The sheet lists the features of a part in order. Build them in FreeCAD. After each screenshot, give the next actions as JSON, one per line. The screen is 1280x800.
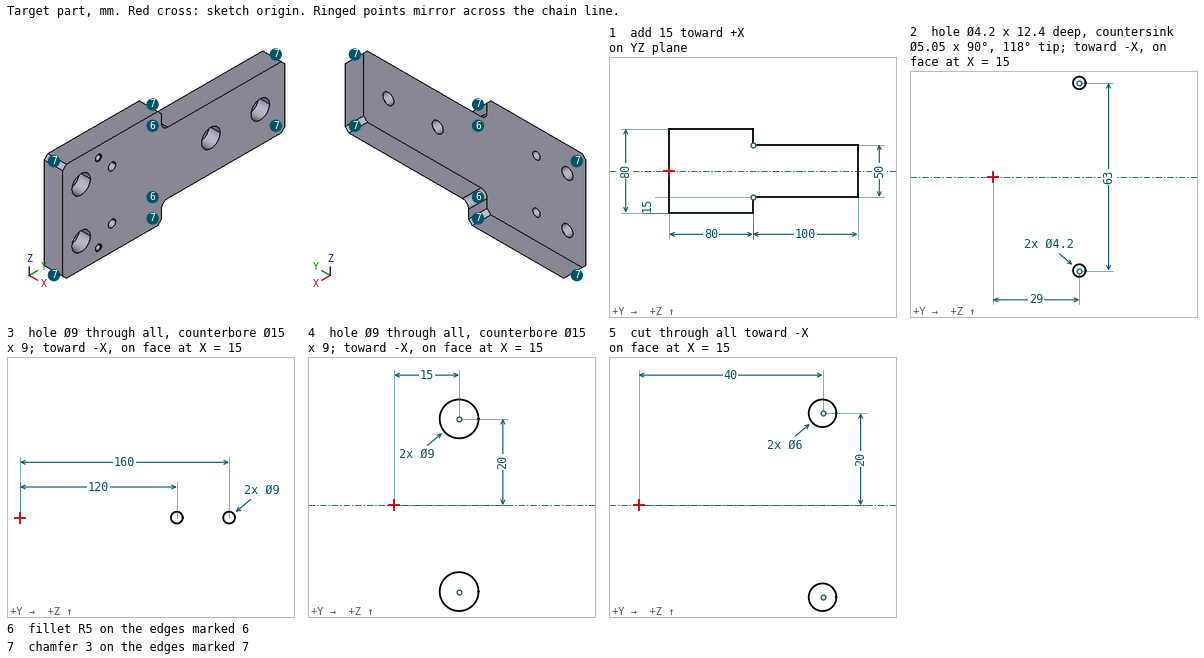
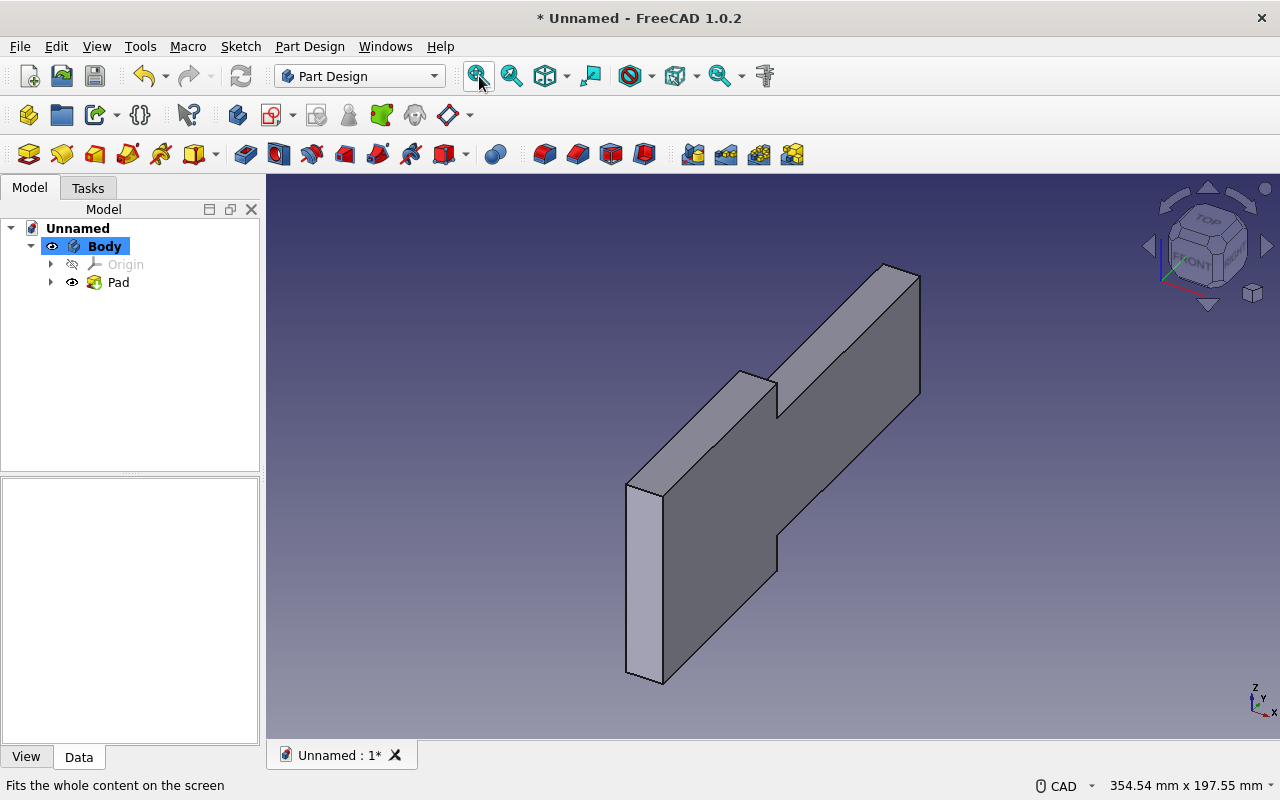
{"action": "left_click", "coordinate": [718, 535]}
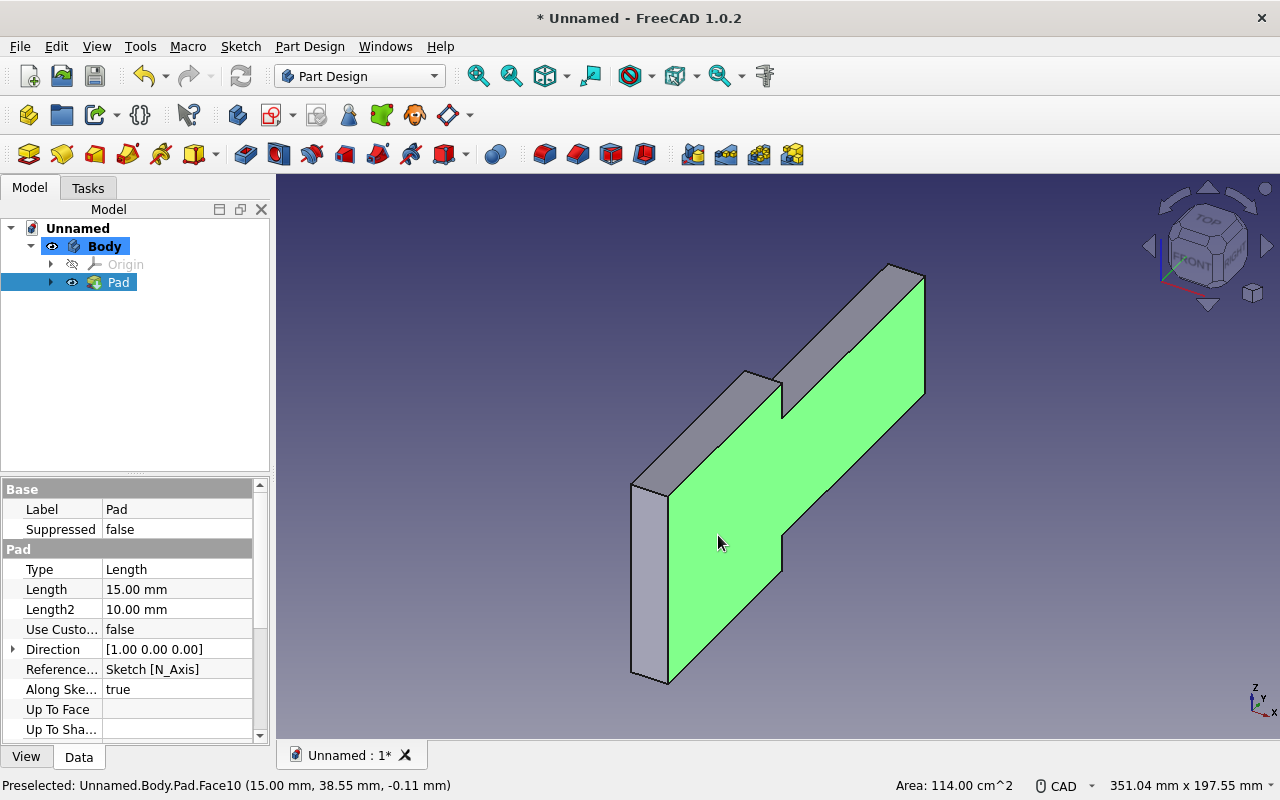
{"action": "left_click", "coordinate": [270, 116]}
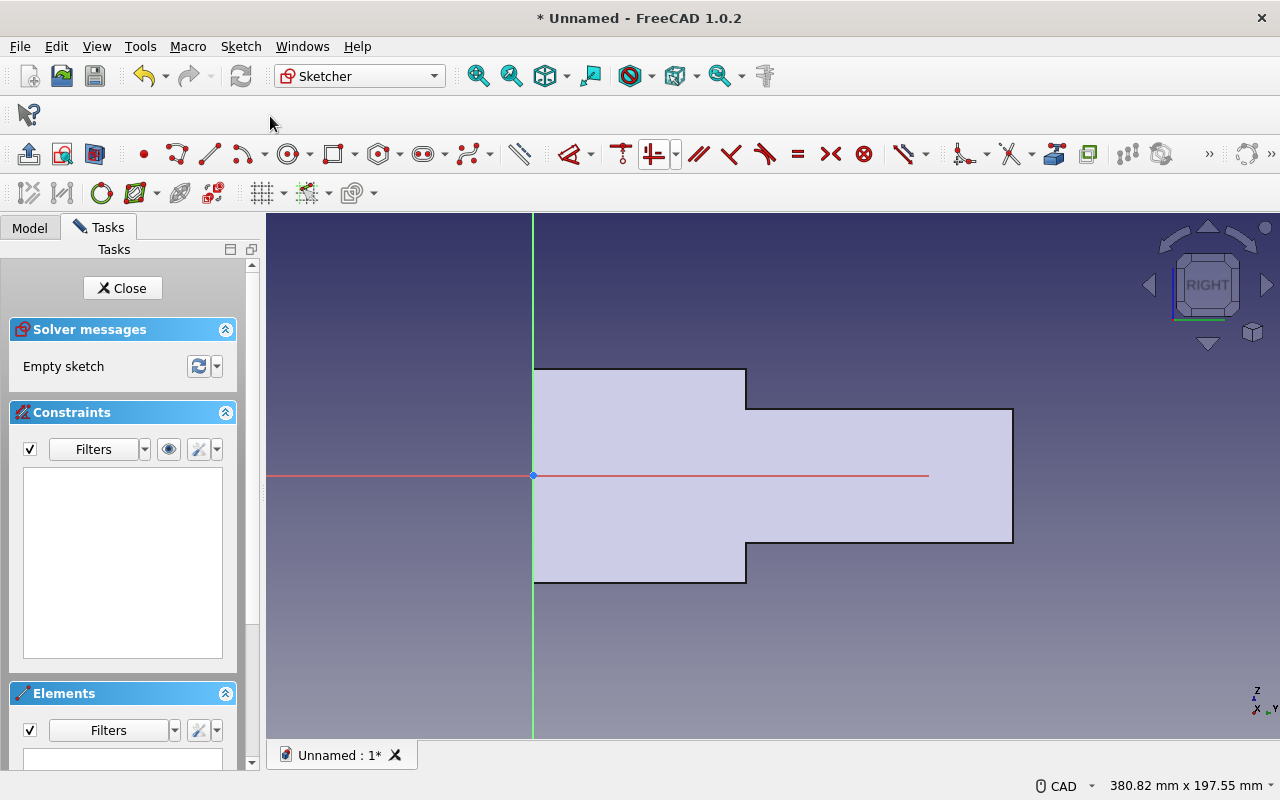
{"action": "scroll", "coordinate": [417, 476], "scroll_direction": "up", "scroll_amount": 3}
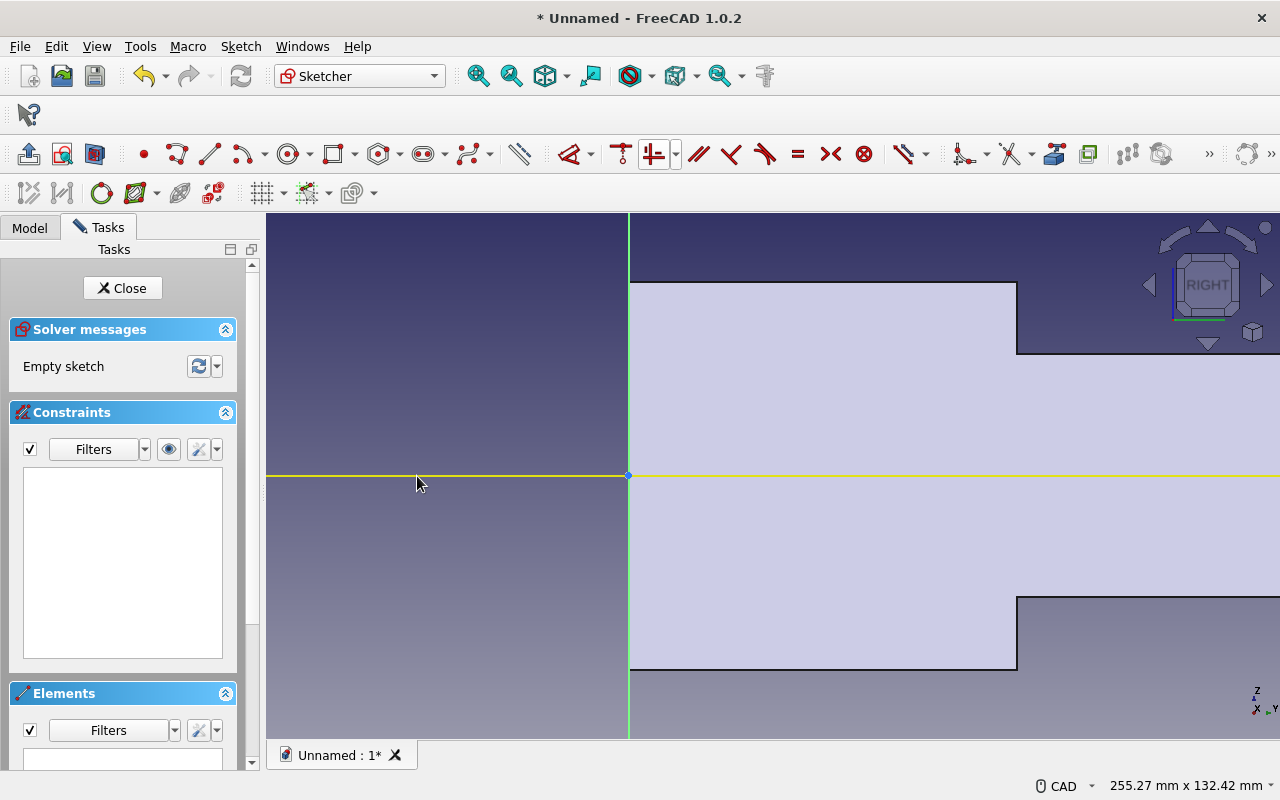
{"action": "left_click", "coordinate": [288, 154]}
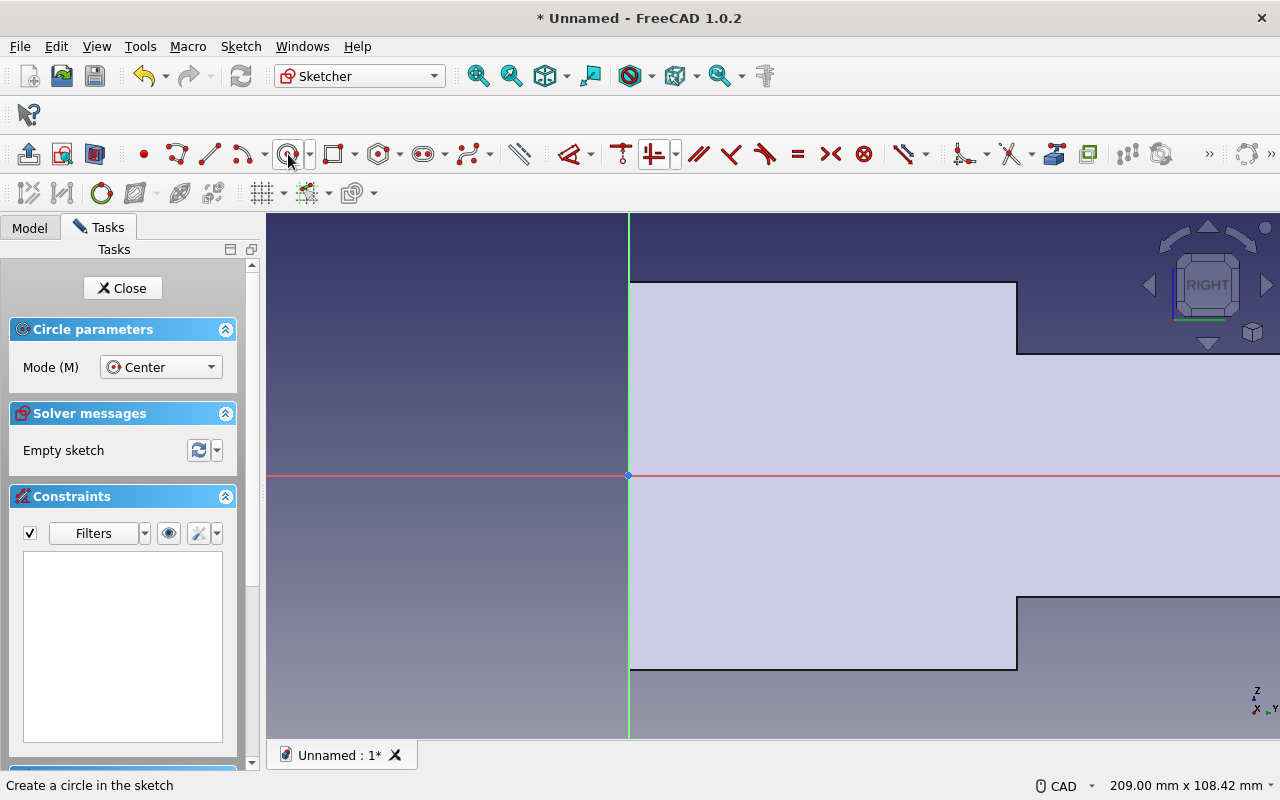
{"action": "scroll", "coordinate": [770, 628], "scroll_direction": "up", "scroll_amount": 5}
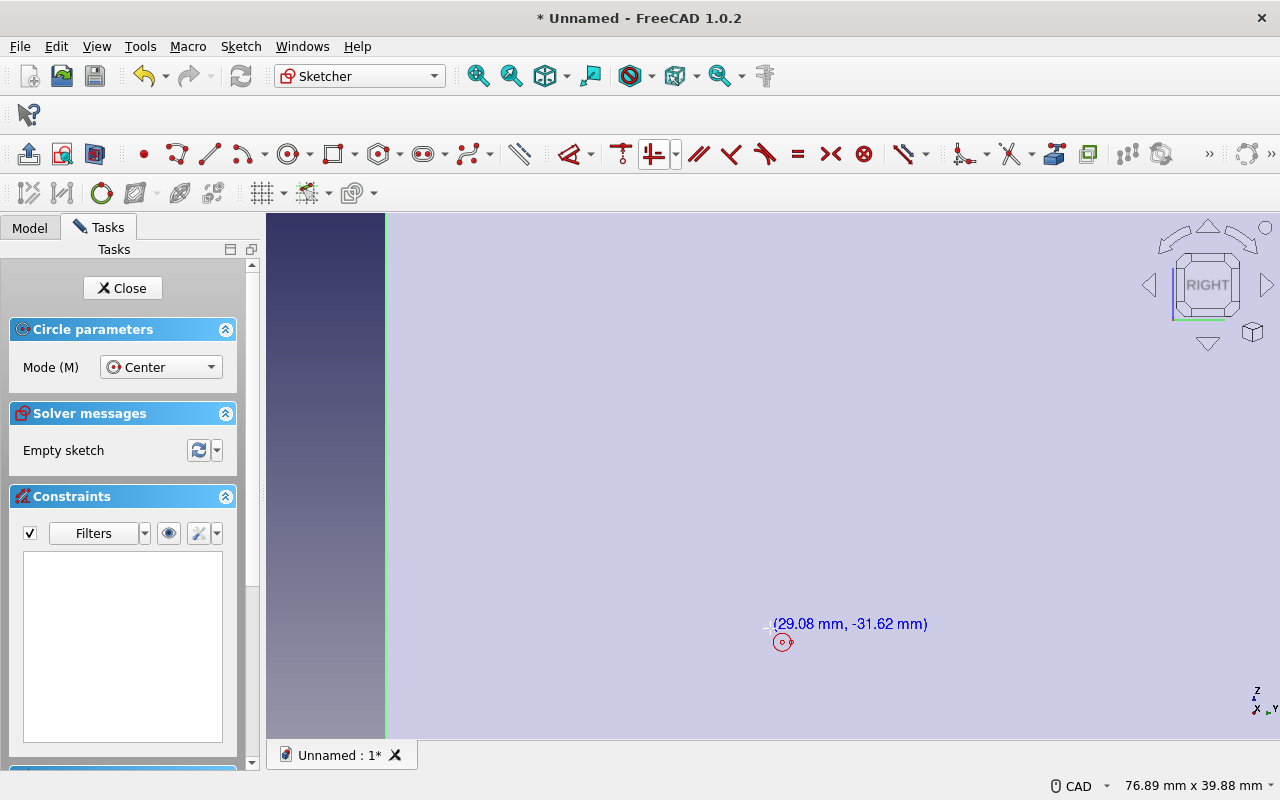
{"action": "left_click", "coordinate": [768, 628]}
{"action": "mouse_move", "coordinate": [788, 608]}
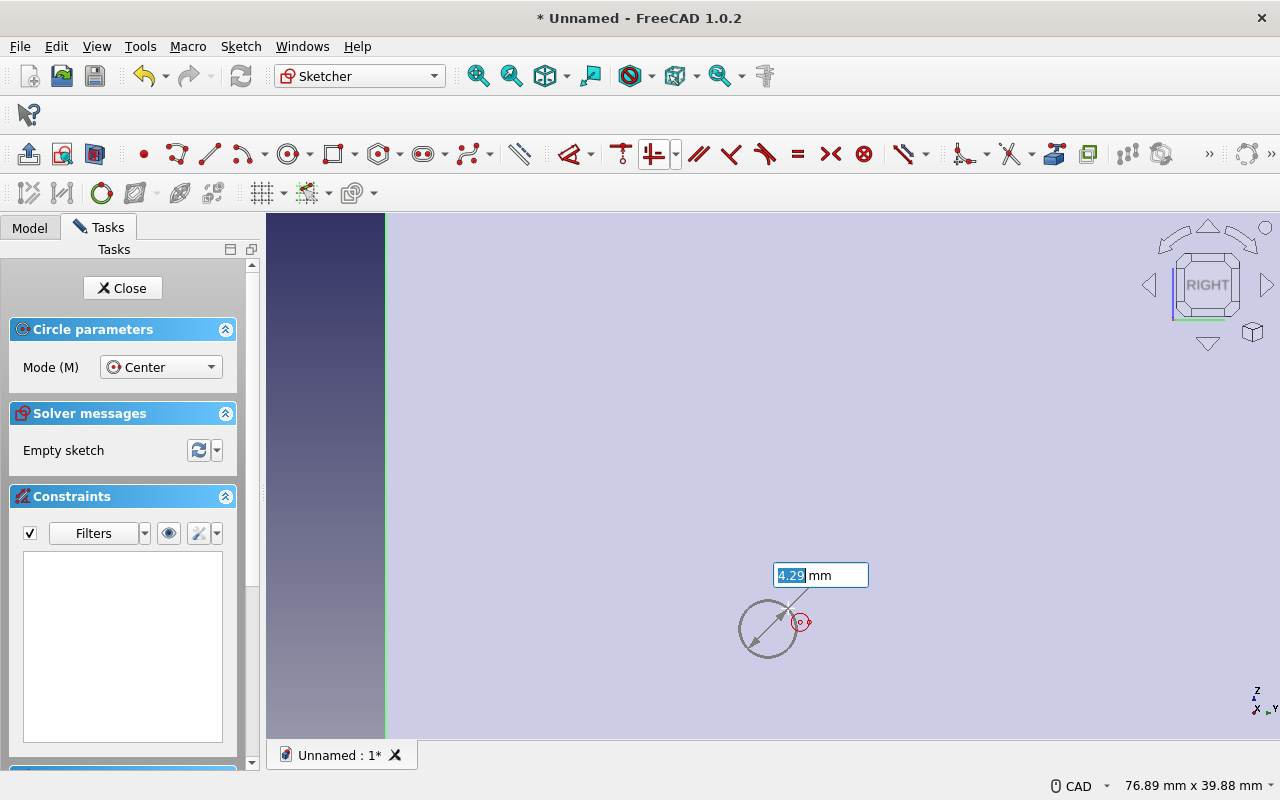
{"action": "type", "text": "4.2"}
{"action": "key", "text": "Return"}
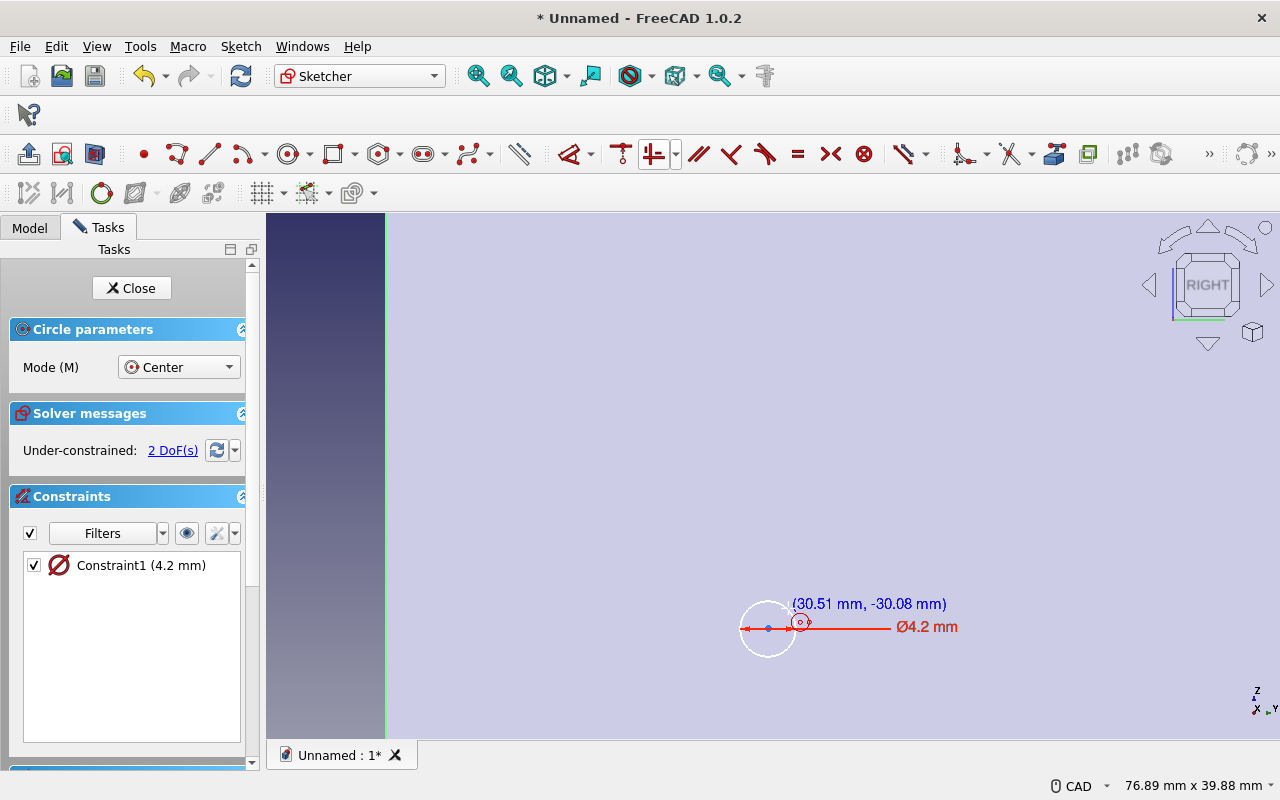
{"action": "scroll", "coordinate": [771, 629], "scroll_direction": "down", "scroll_amount": 5}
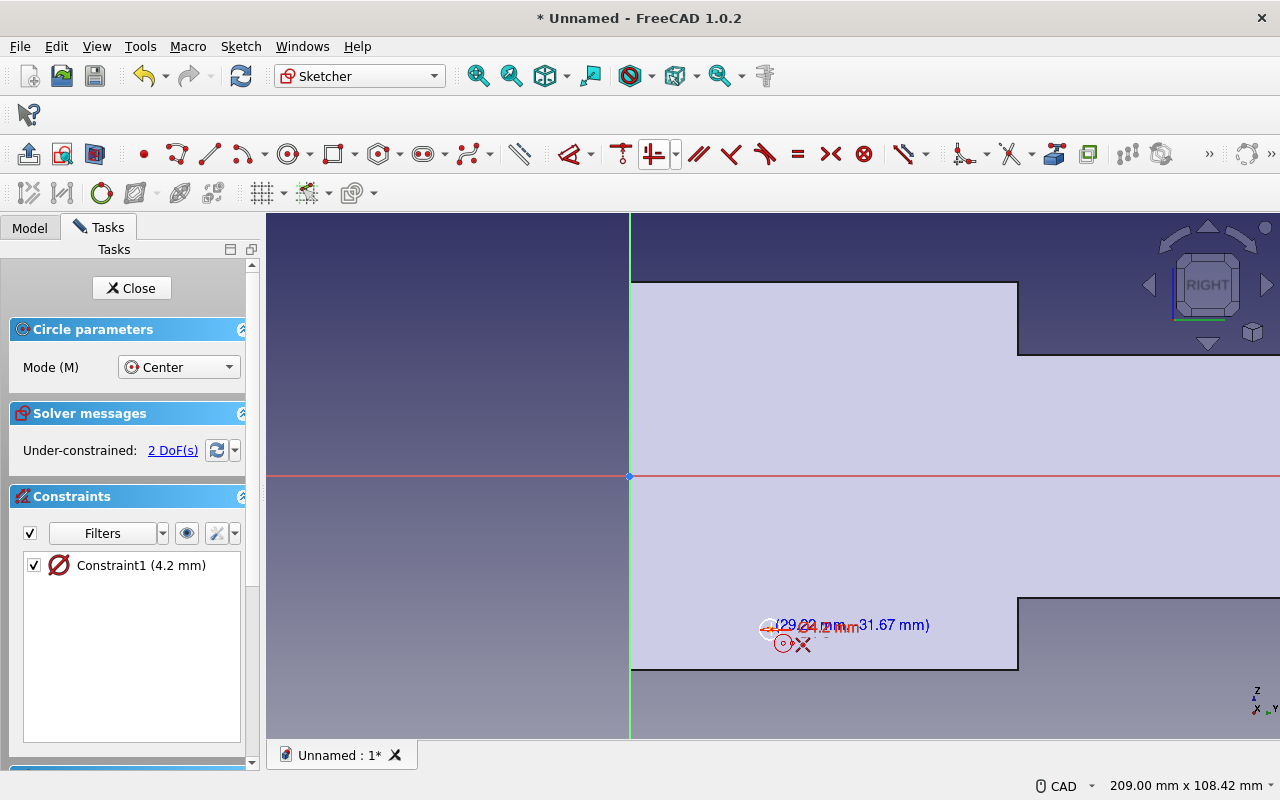
{"action": "scroll", "coordinate": [770, 323], "scroll_direction": "up", "scroll_amount": 5}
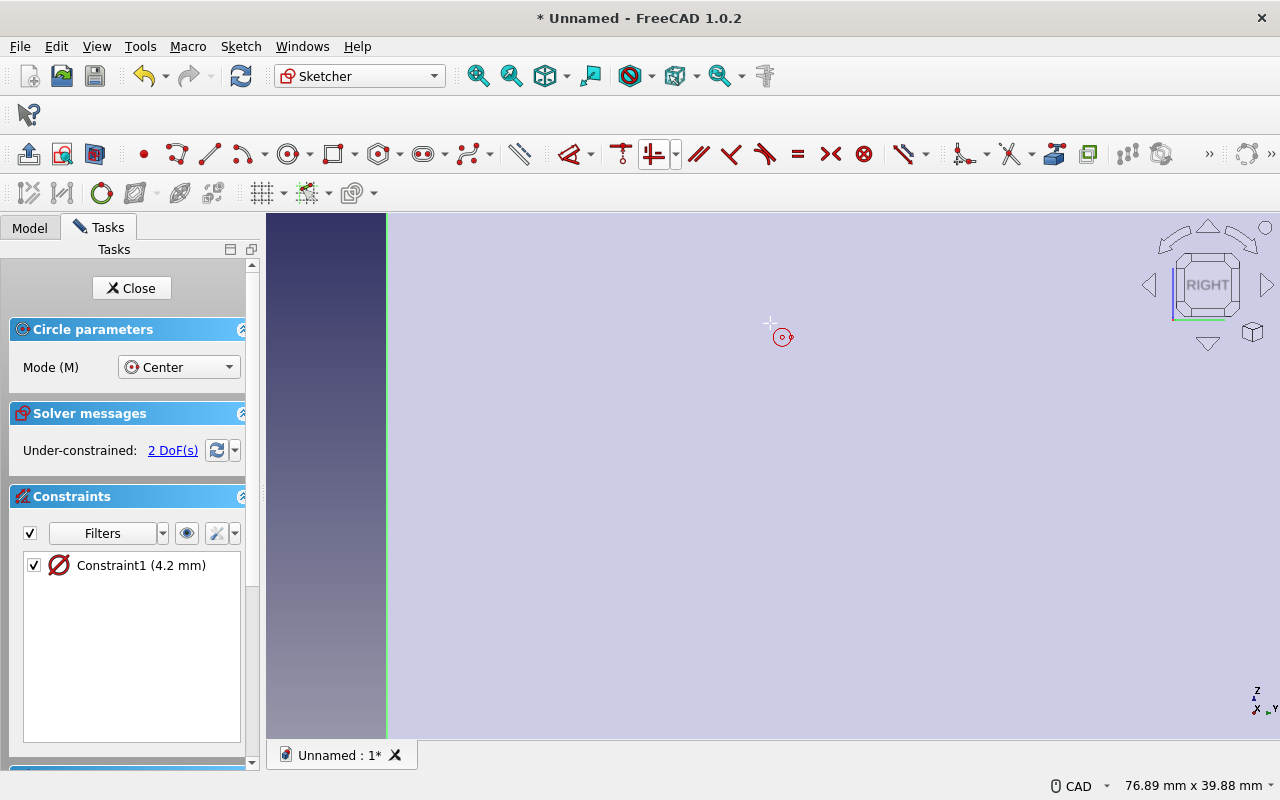
{"action": "left_click", "coordinate": [770, 324]}
{"action": "mouse_move", "coordinate": [789, 304]}